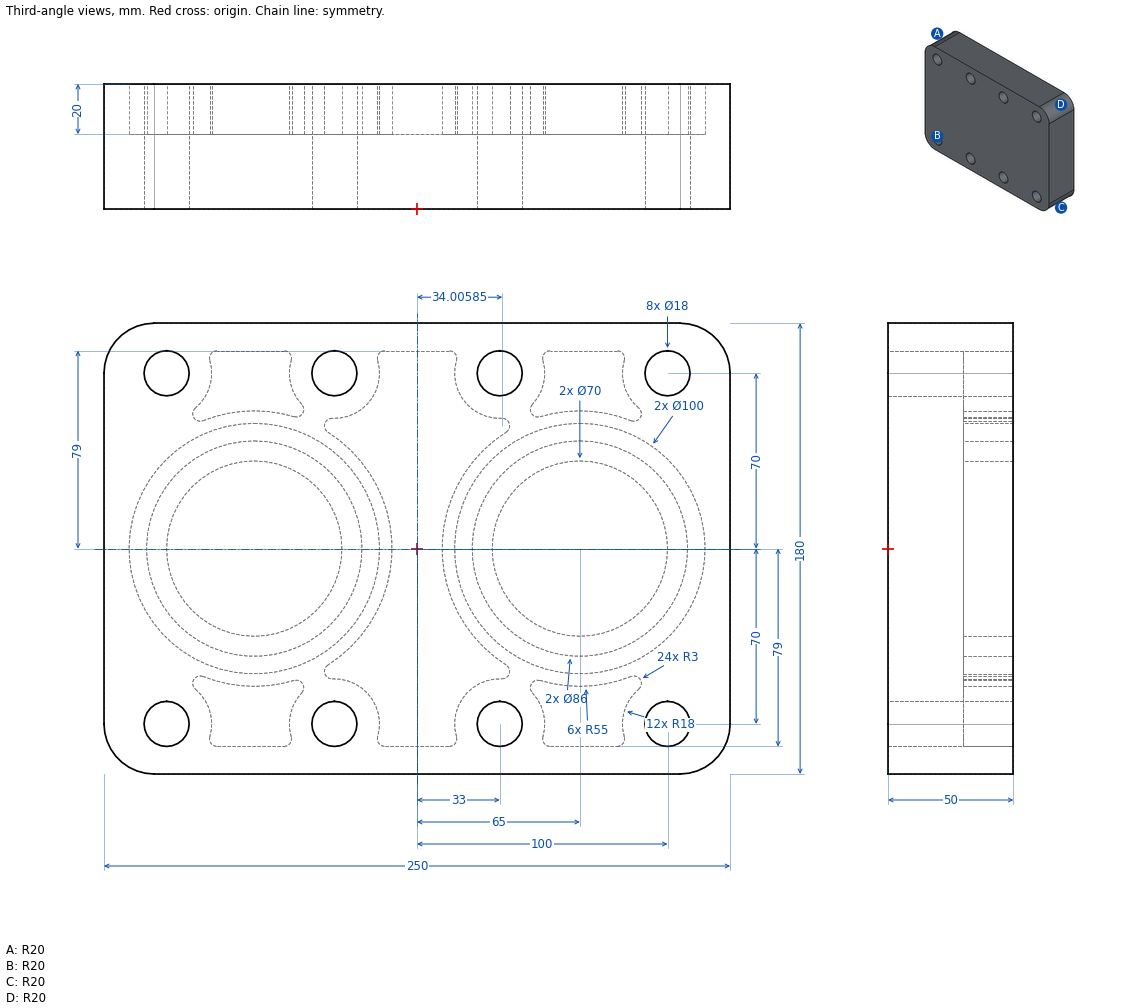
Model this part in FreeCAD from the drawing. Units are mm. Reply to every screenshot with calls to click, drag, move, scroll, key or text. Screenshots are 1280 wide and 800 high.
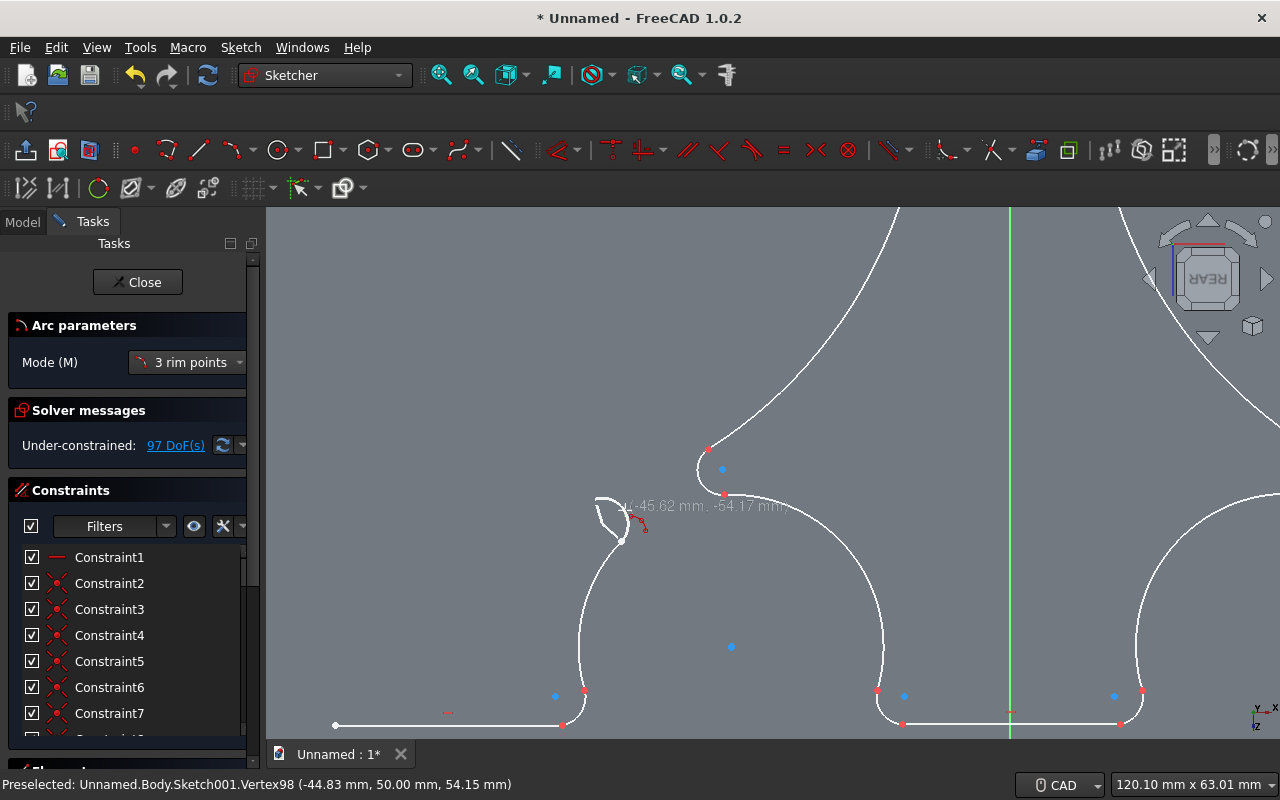
click(625, 509)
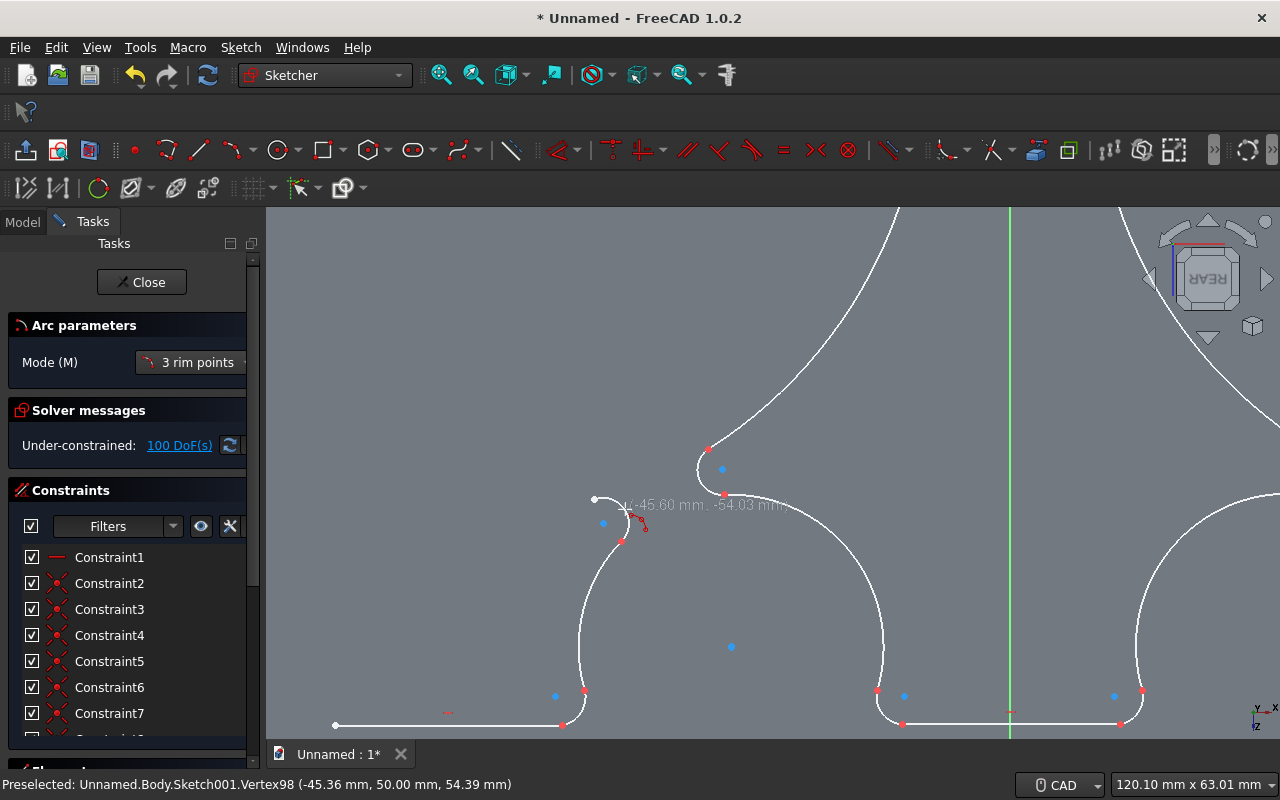
click(595, 499)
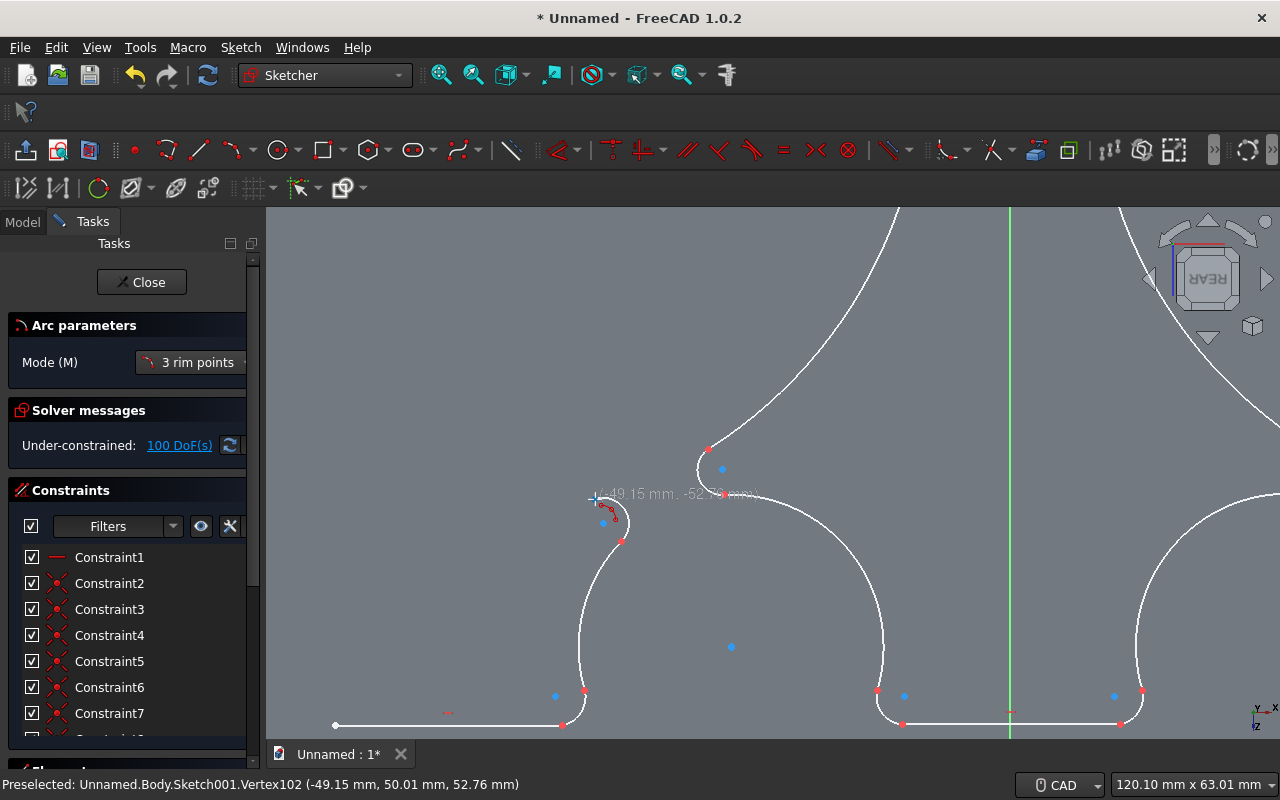
scroll(605, 610, down, 7)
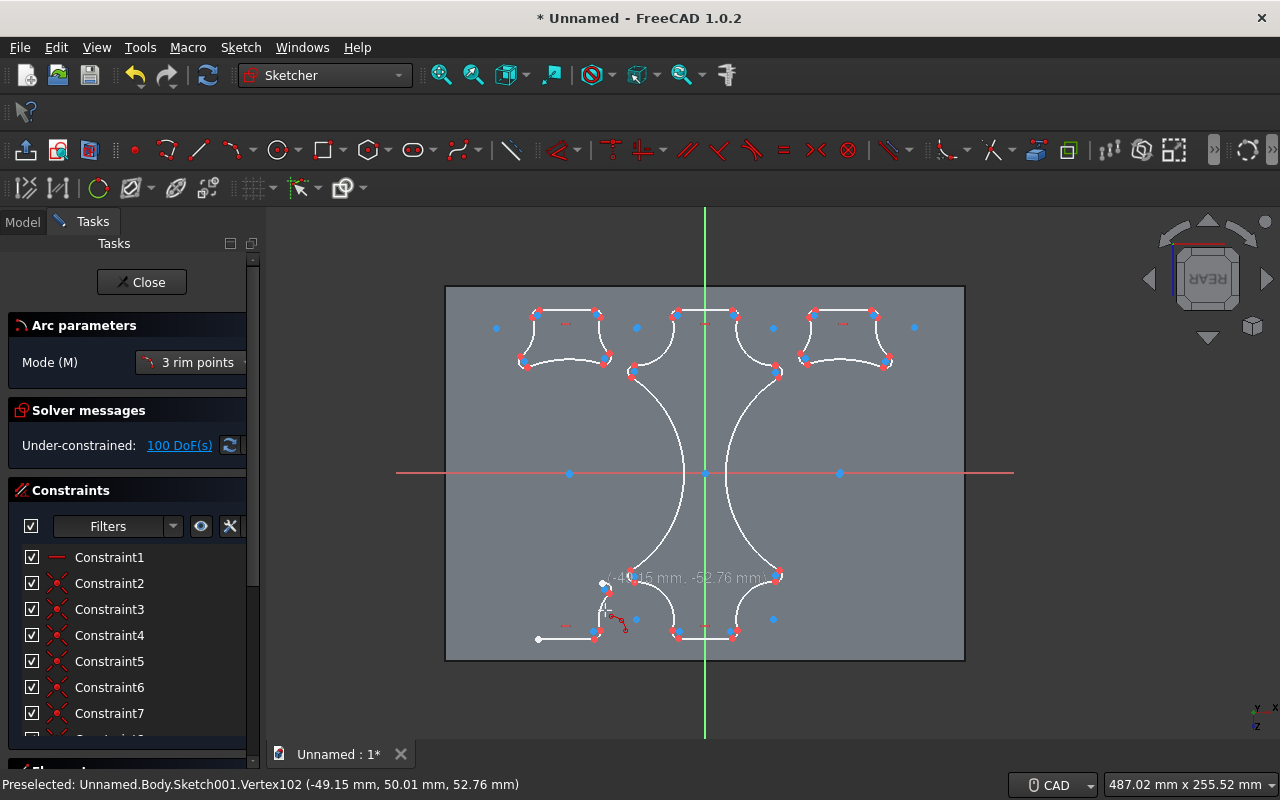
click(527, 580)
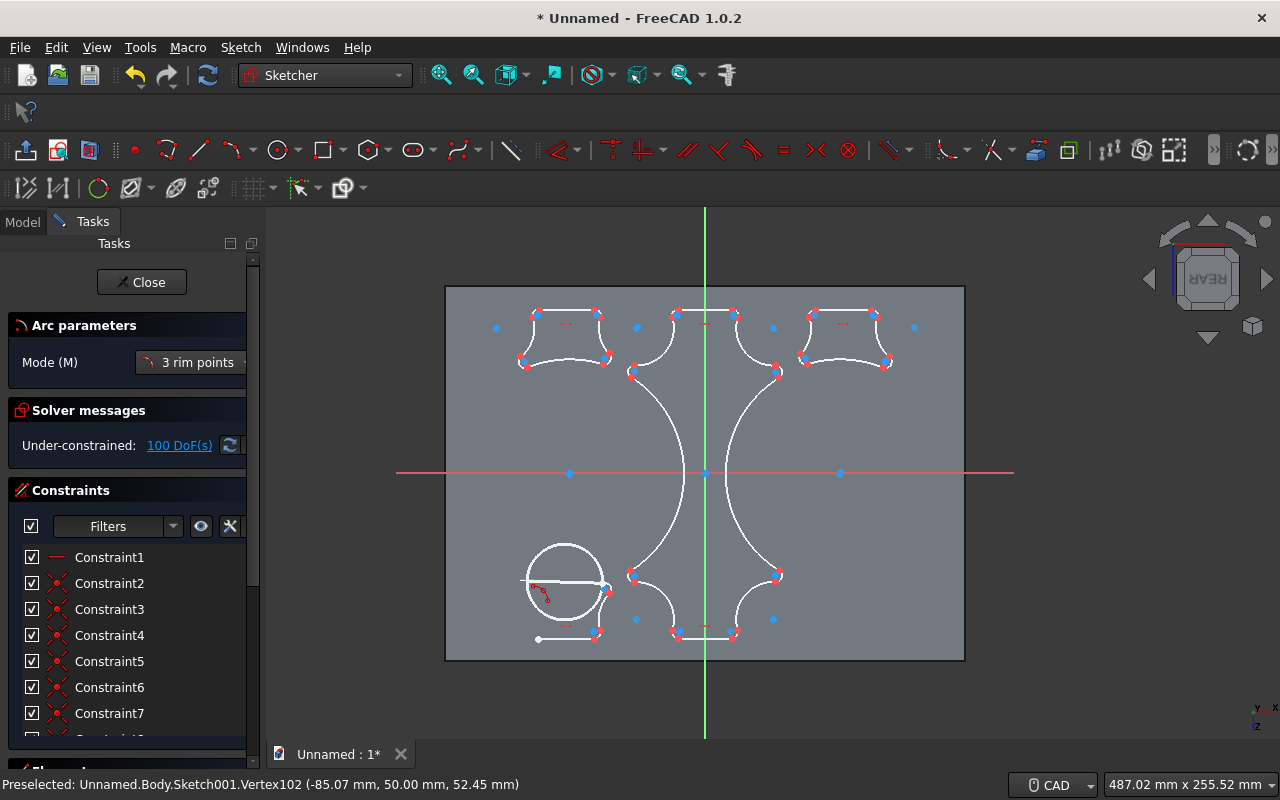
scroll(565, 588, up, 5)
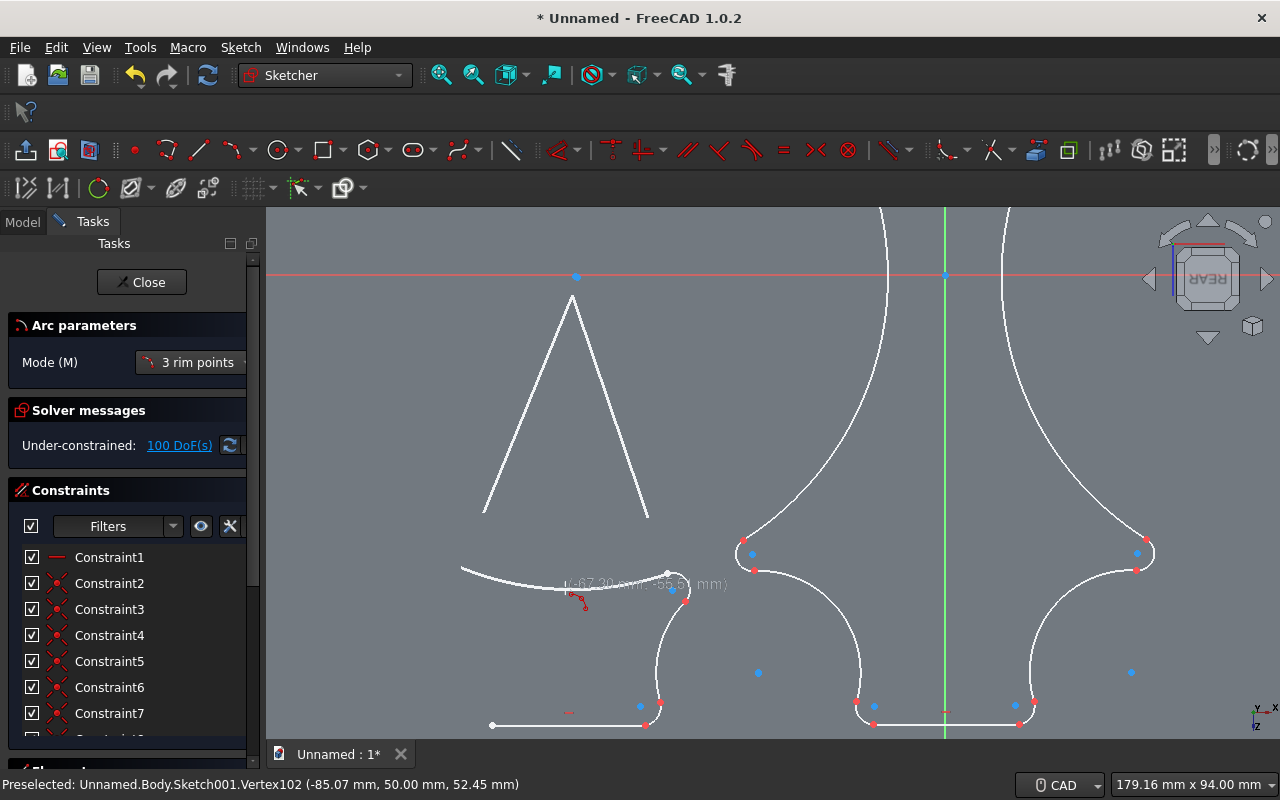
click(564, 586)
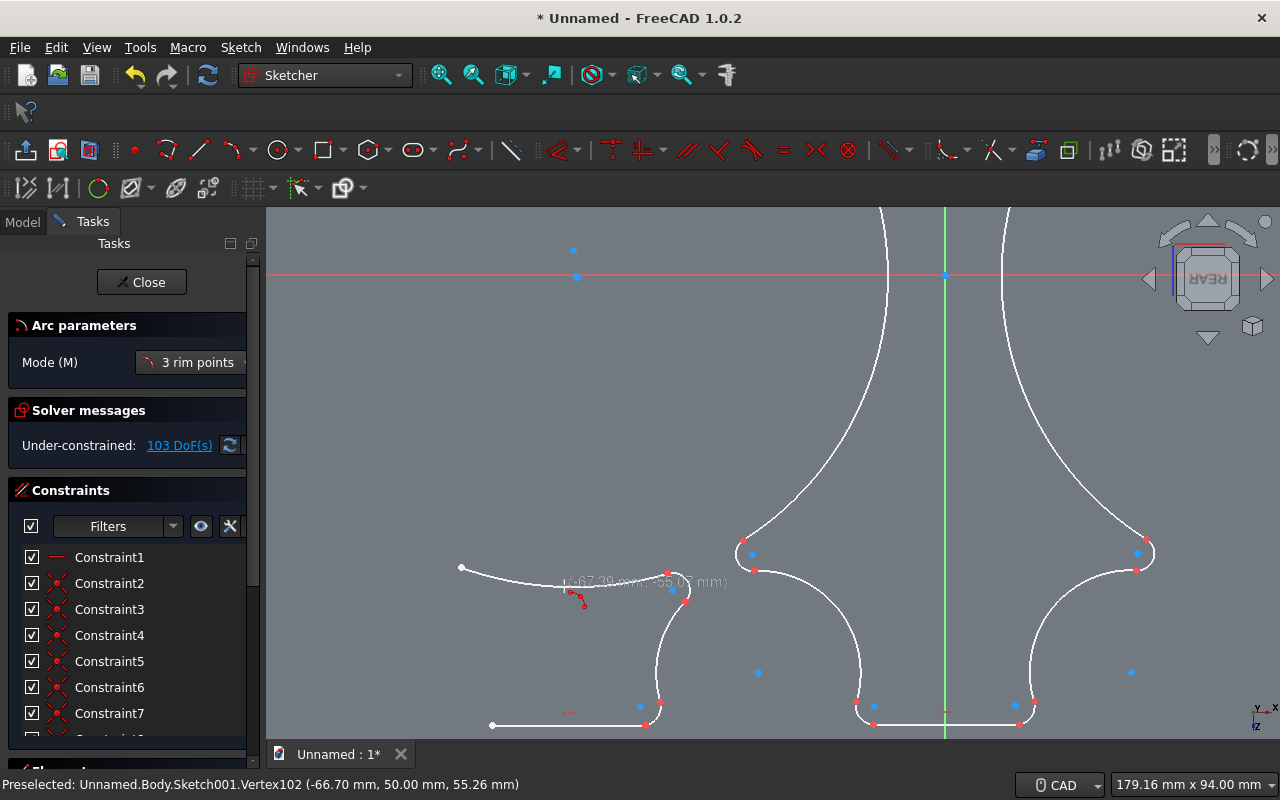
click(461, 568)
click(444, 593)
click(441, 571)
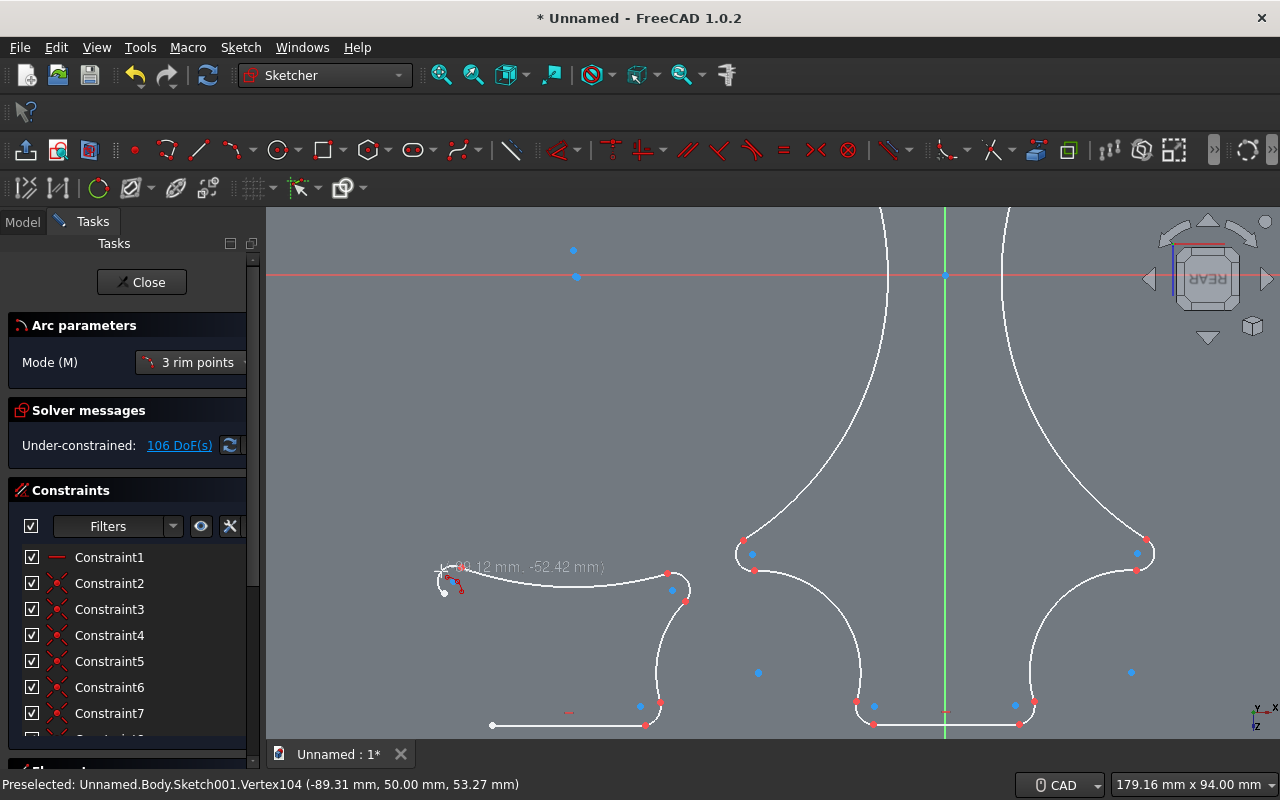
click(444, 594)
click(477, 701)
click(477, 642)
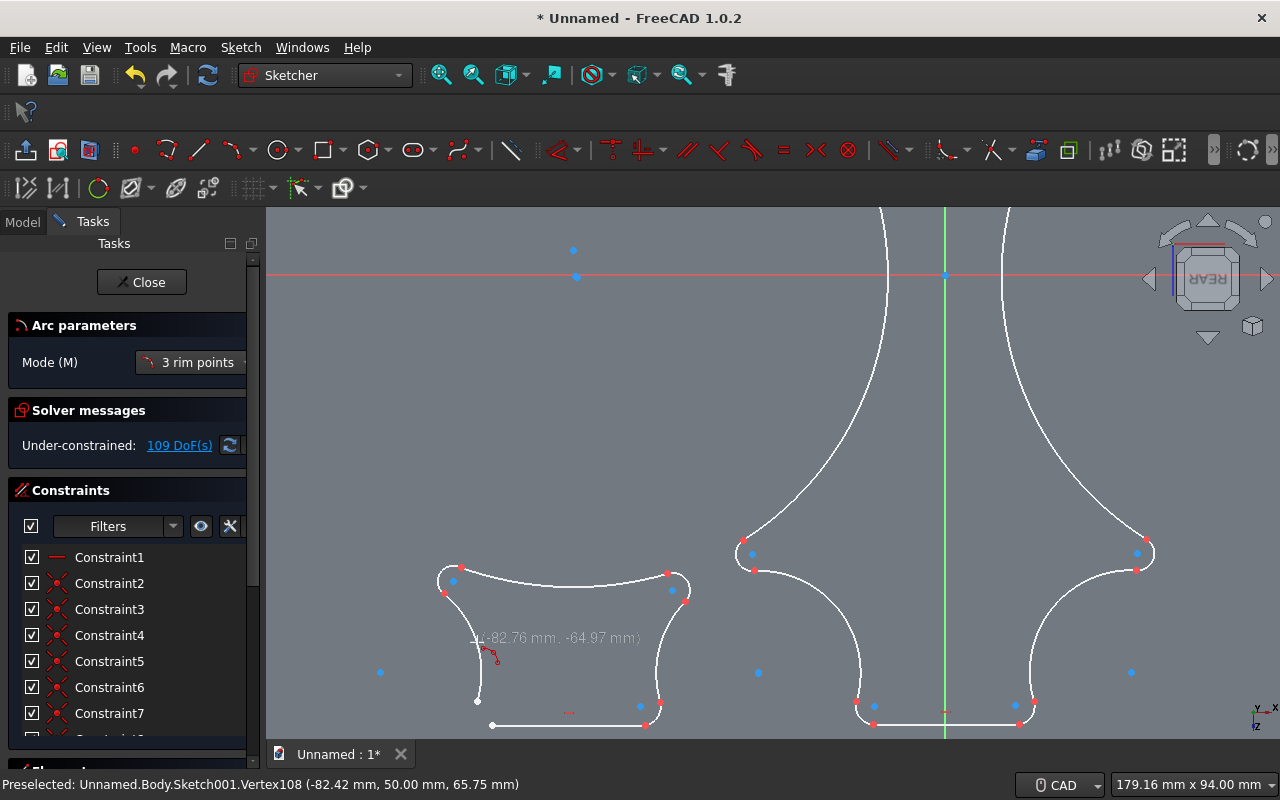
click(477, 702)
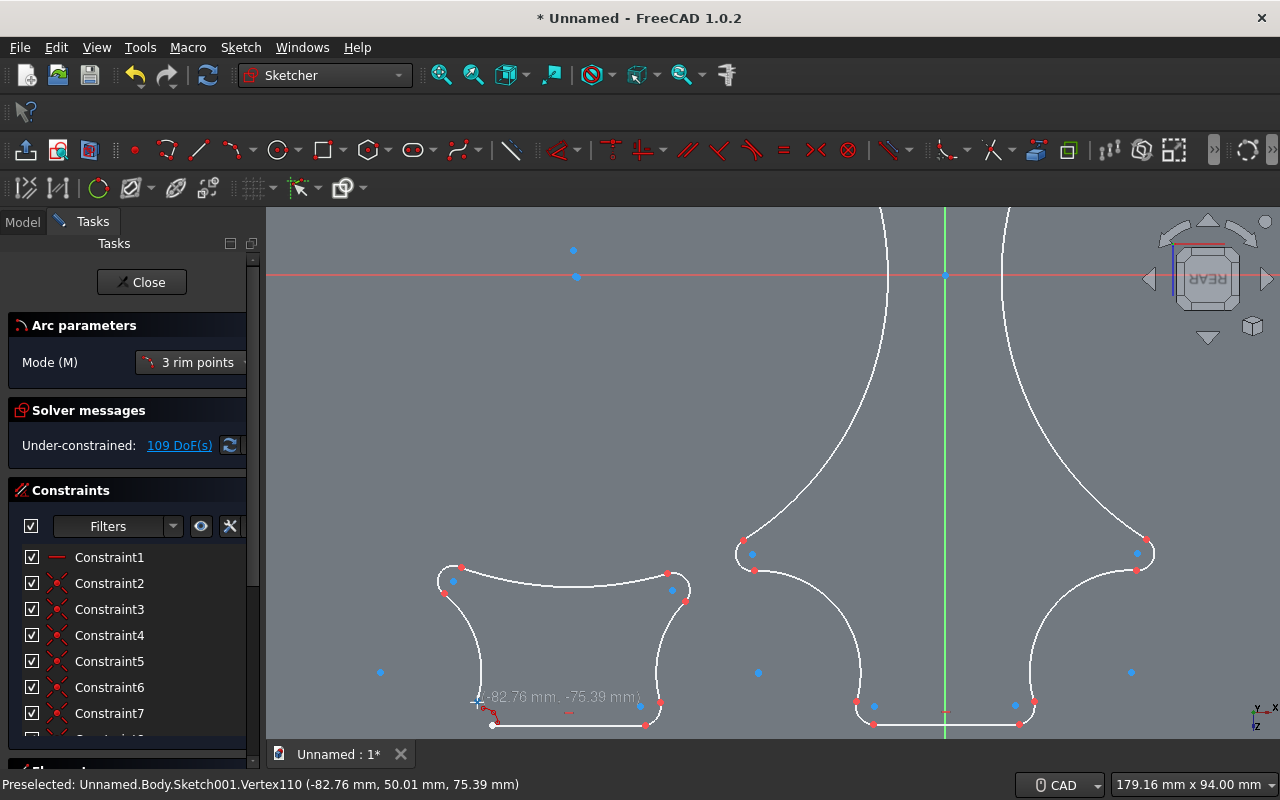
scroll(564, 588, down, 5)